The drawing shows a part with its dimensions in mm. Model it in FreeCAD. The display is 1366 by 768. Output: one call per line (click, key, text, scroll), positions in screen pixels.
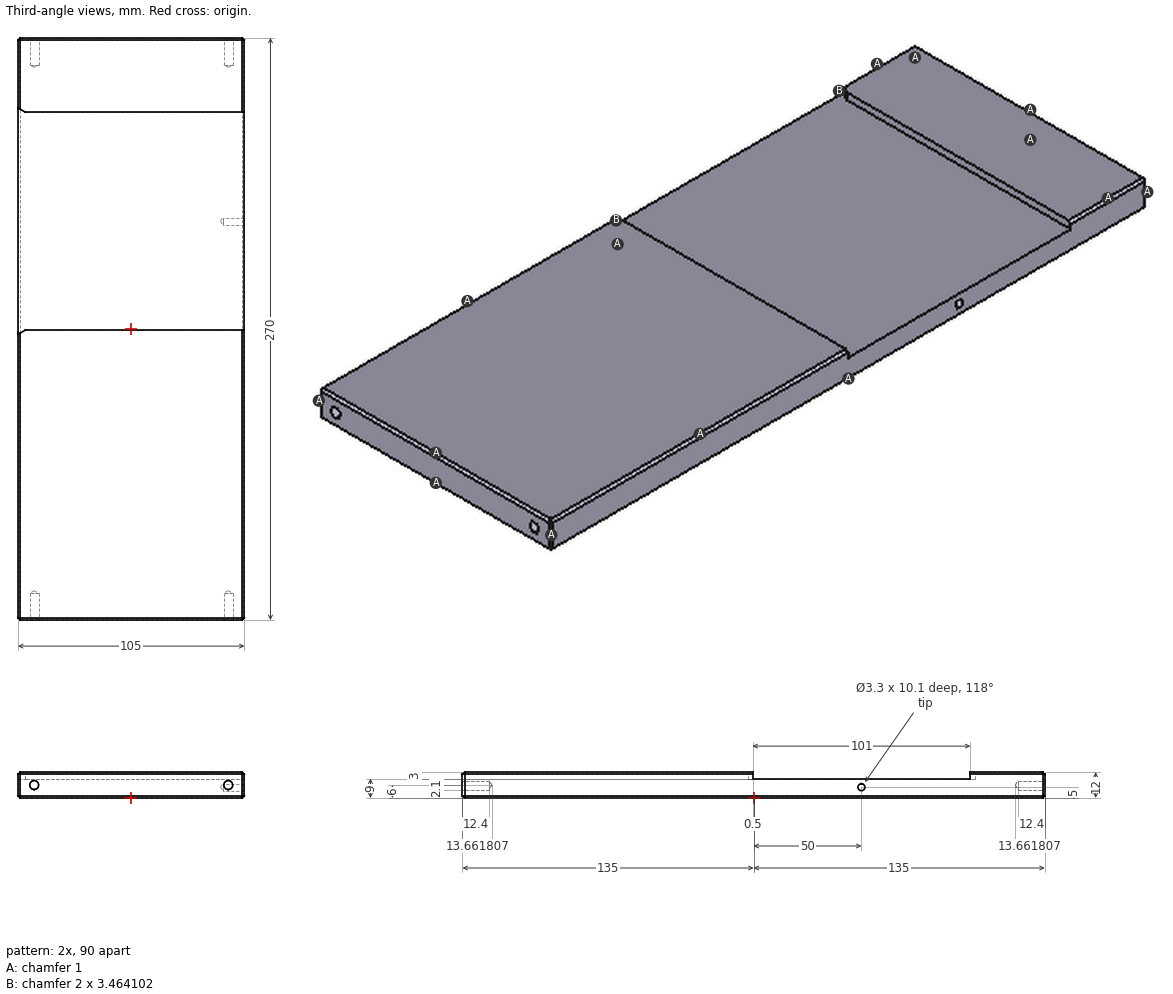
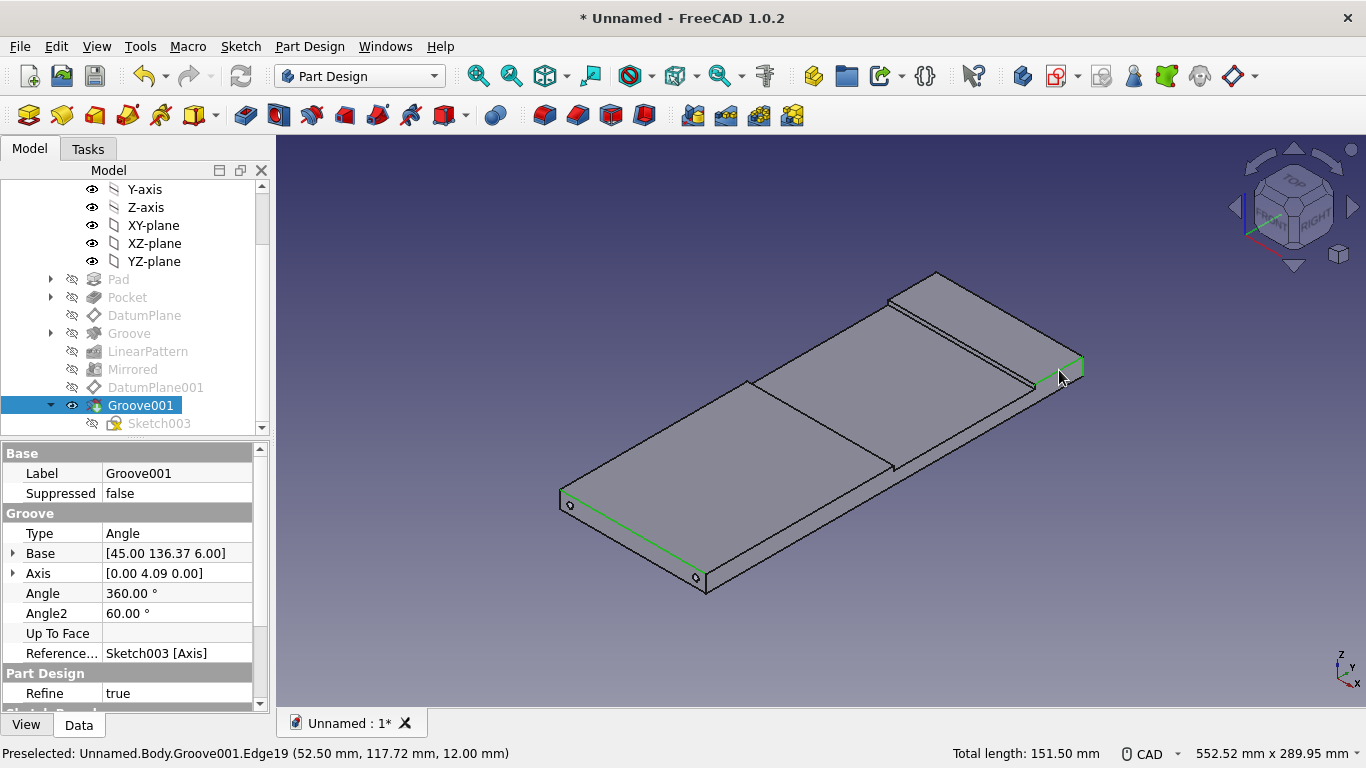
click(800, 519, ctrl)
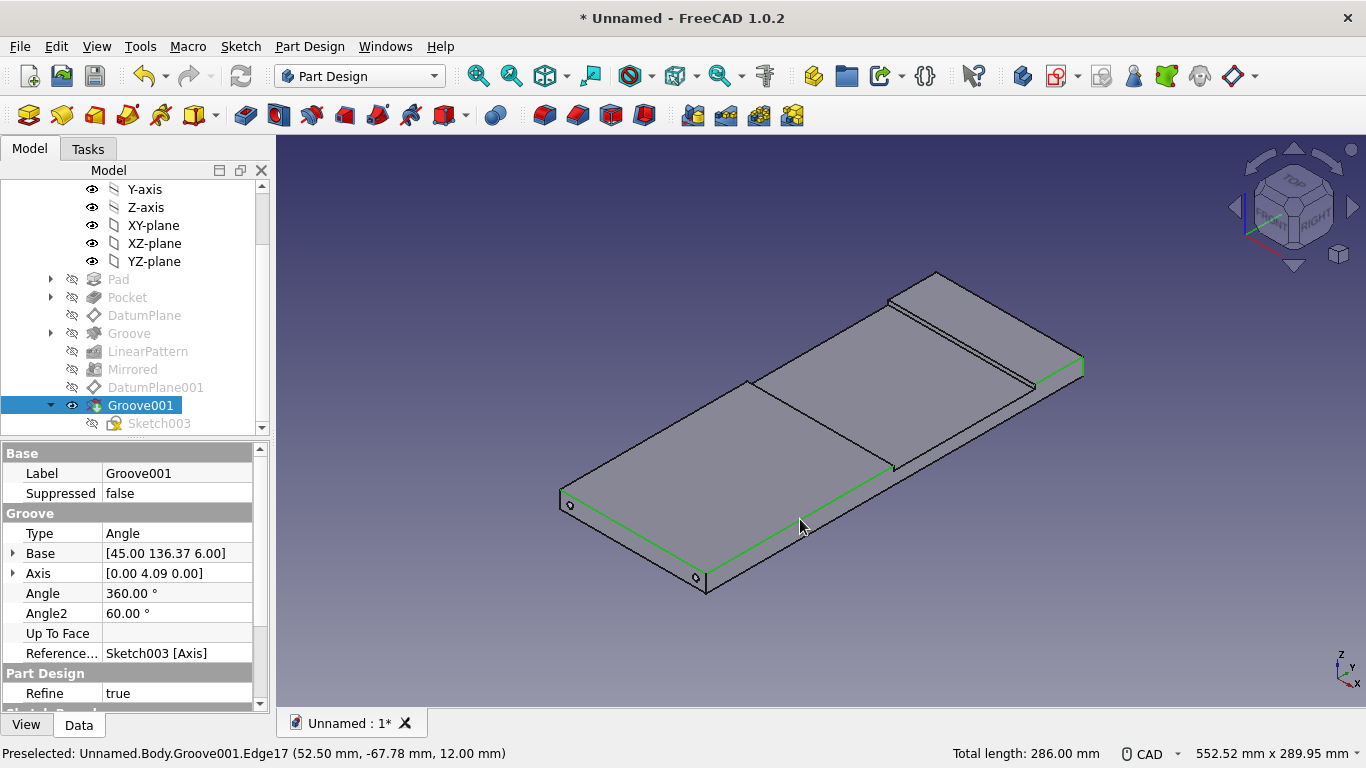
click(706, 583, ctrl)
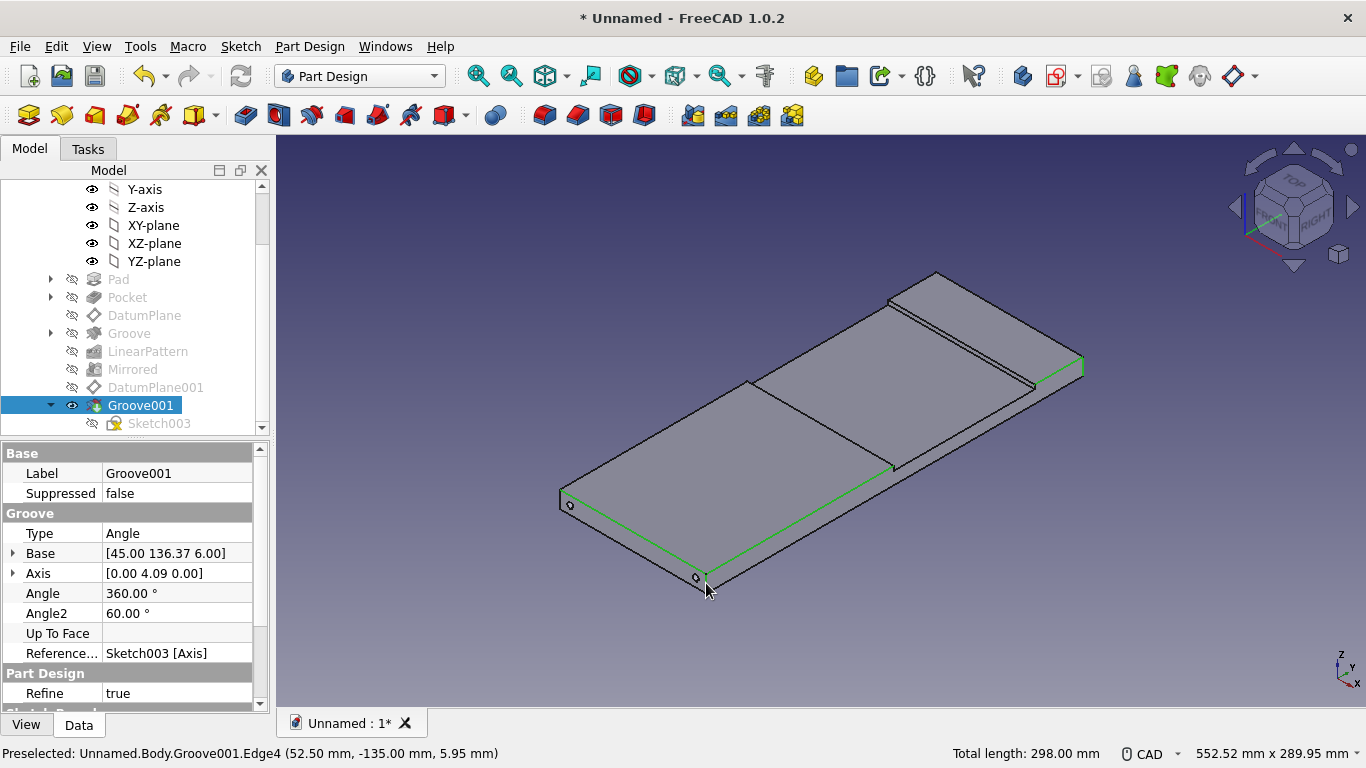
key(2)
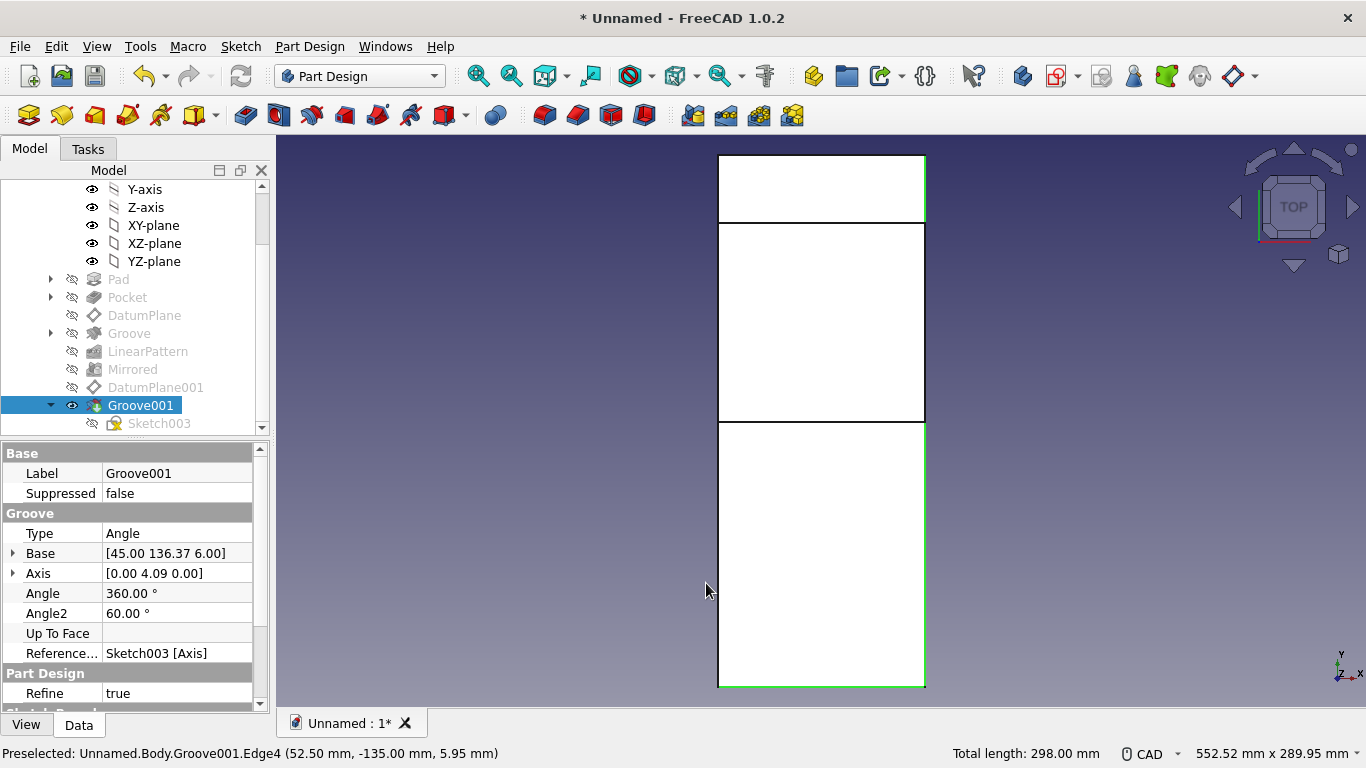
click(718, 188, ctrl)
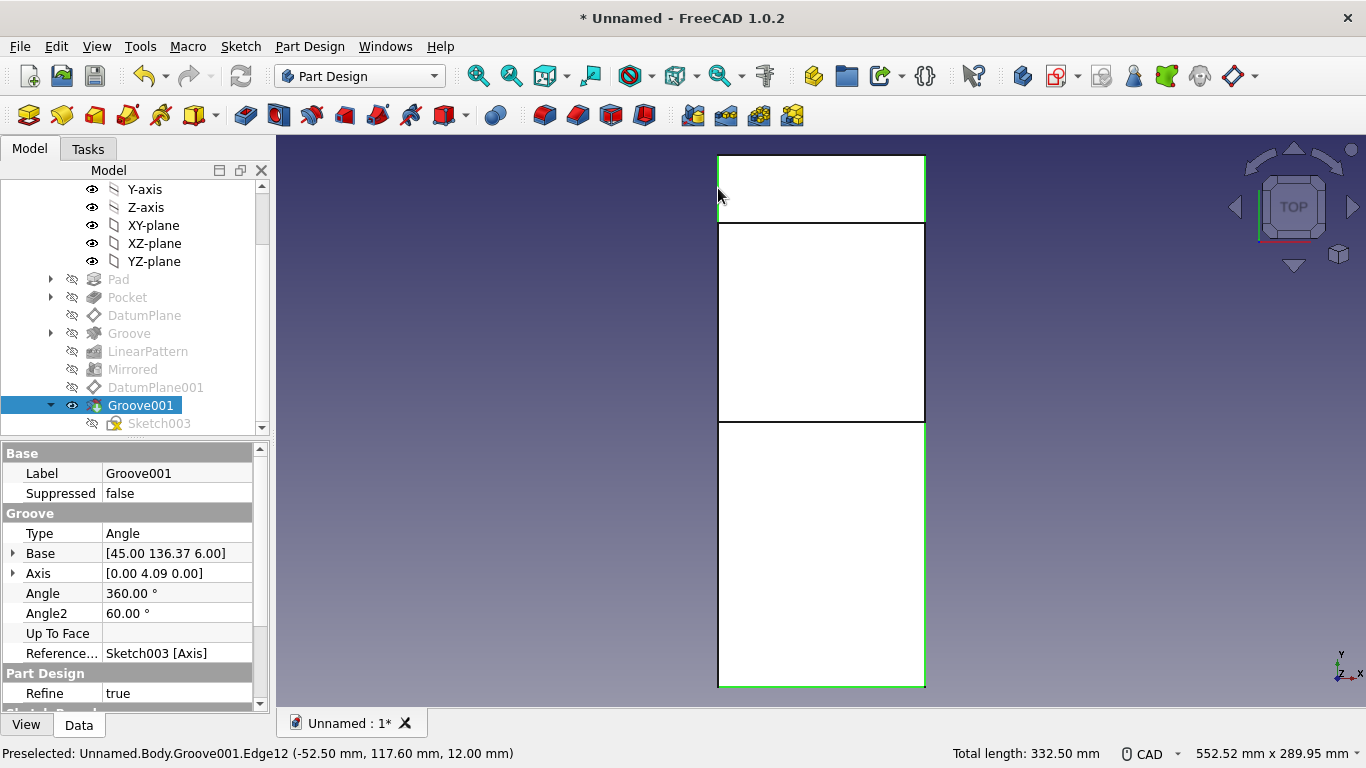
click(718, 554, ctrl)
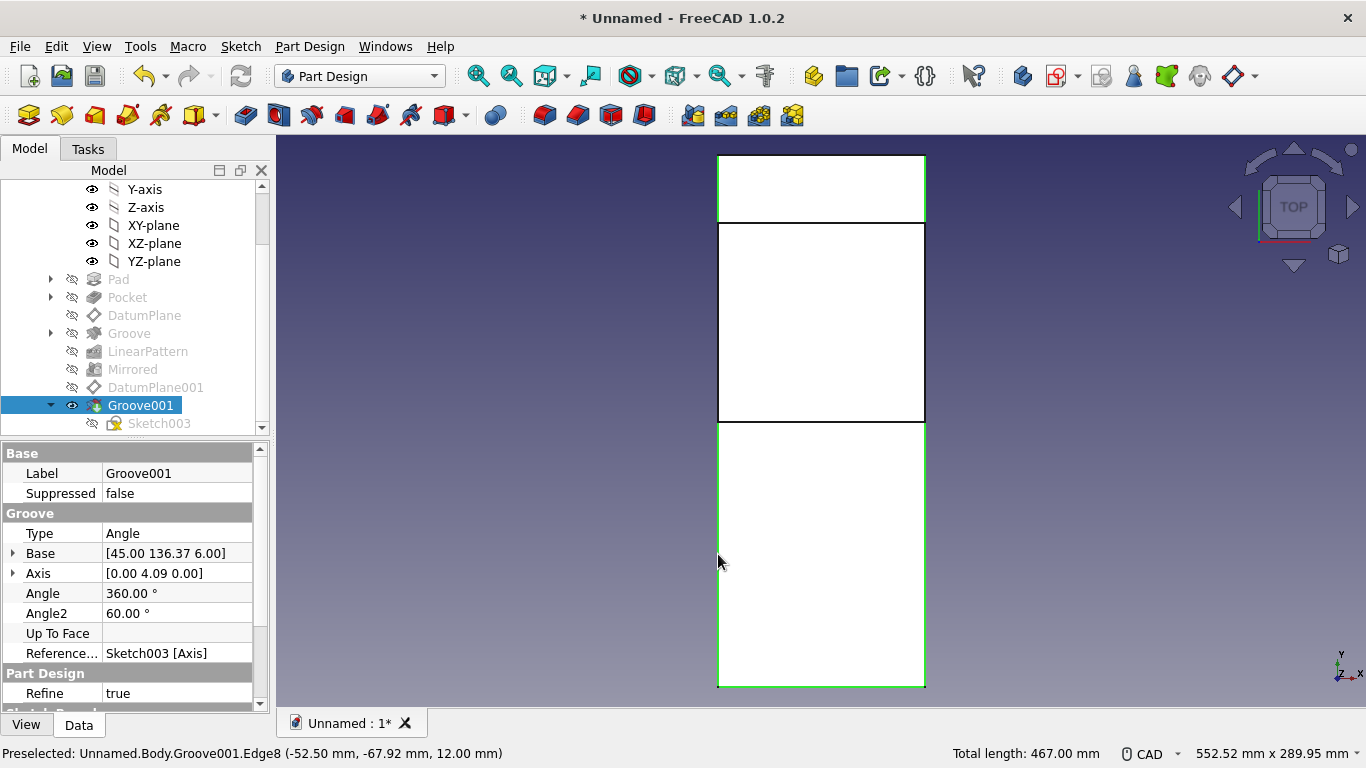
key(1)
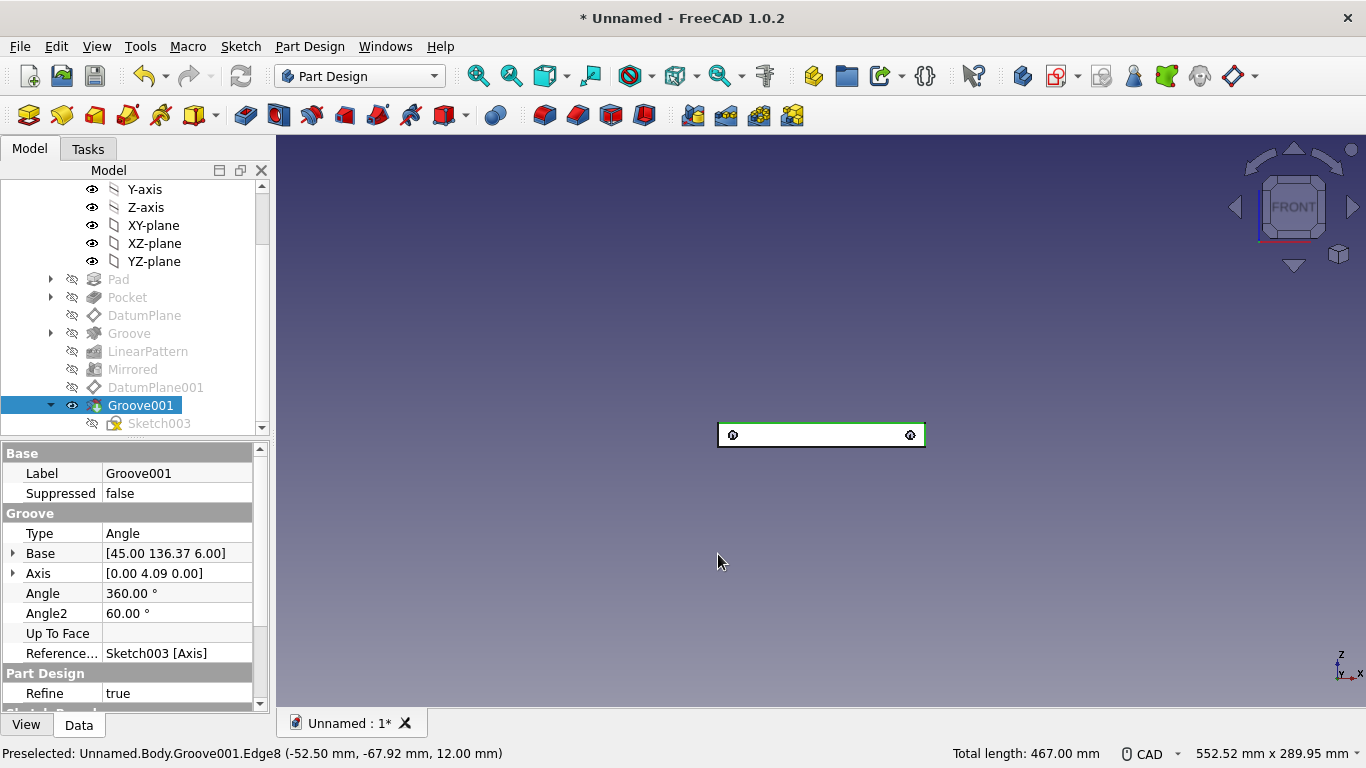
click(479, 76)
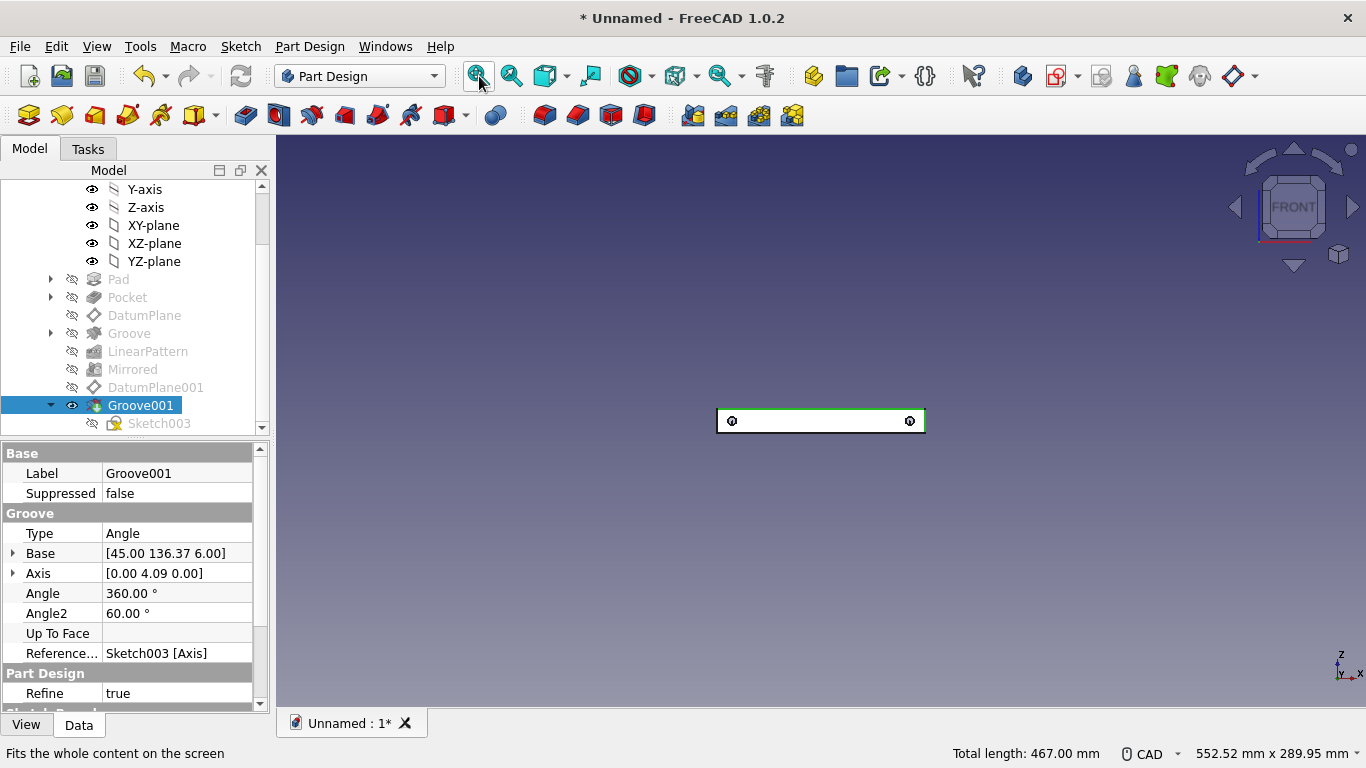
click(717, 420, ctrl)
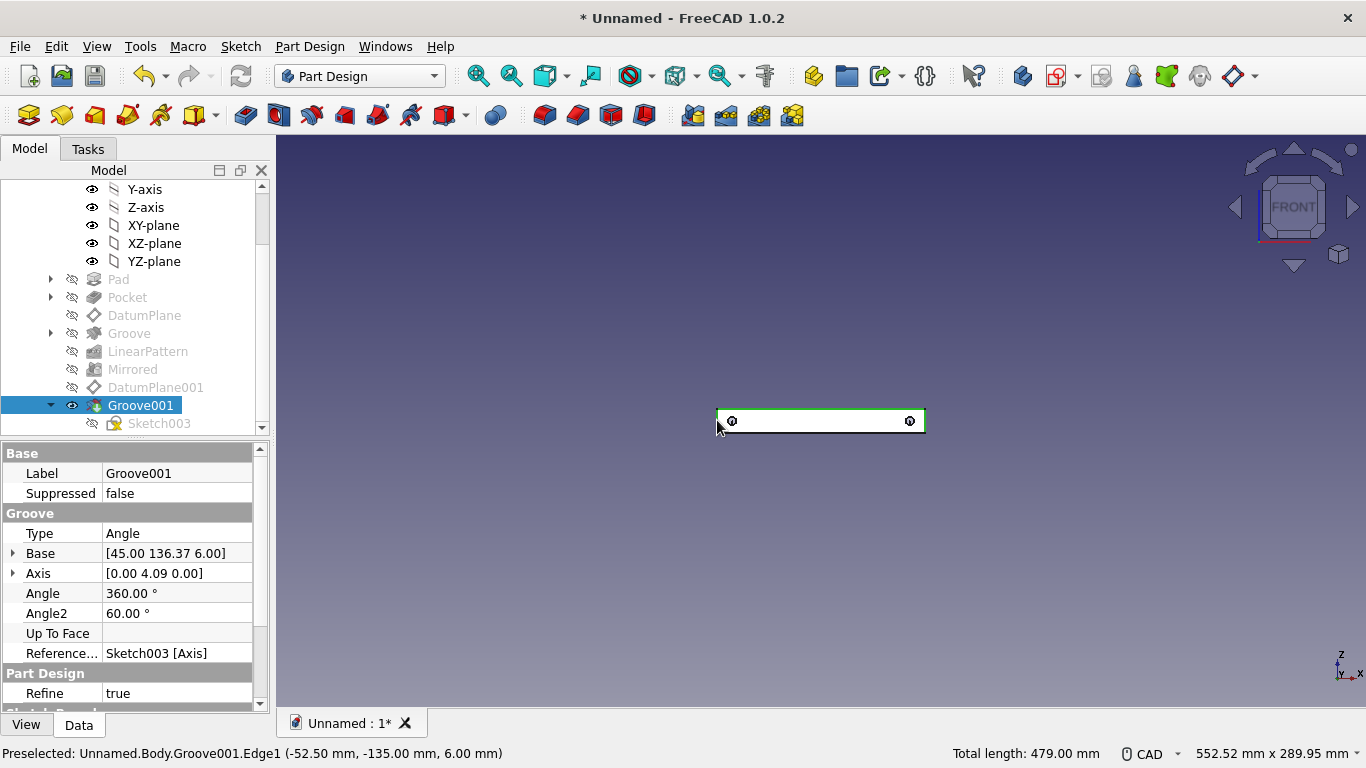
key(3)